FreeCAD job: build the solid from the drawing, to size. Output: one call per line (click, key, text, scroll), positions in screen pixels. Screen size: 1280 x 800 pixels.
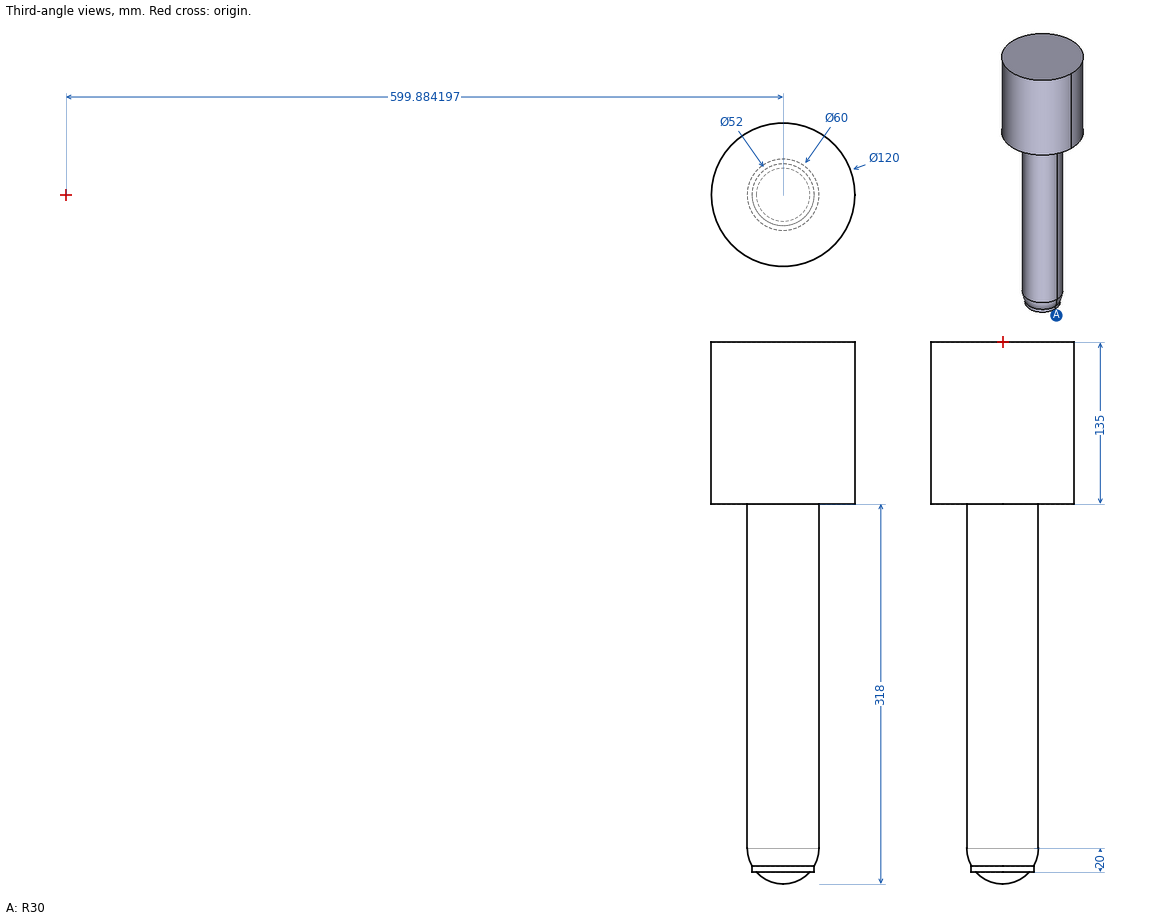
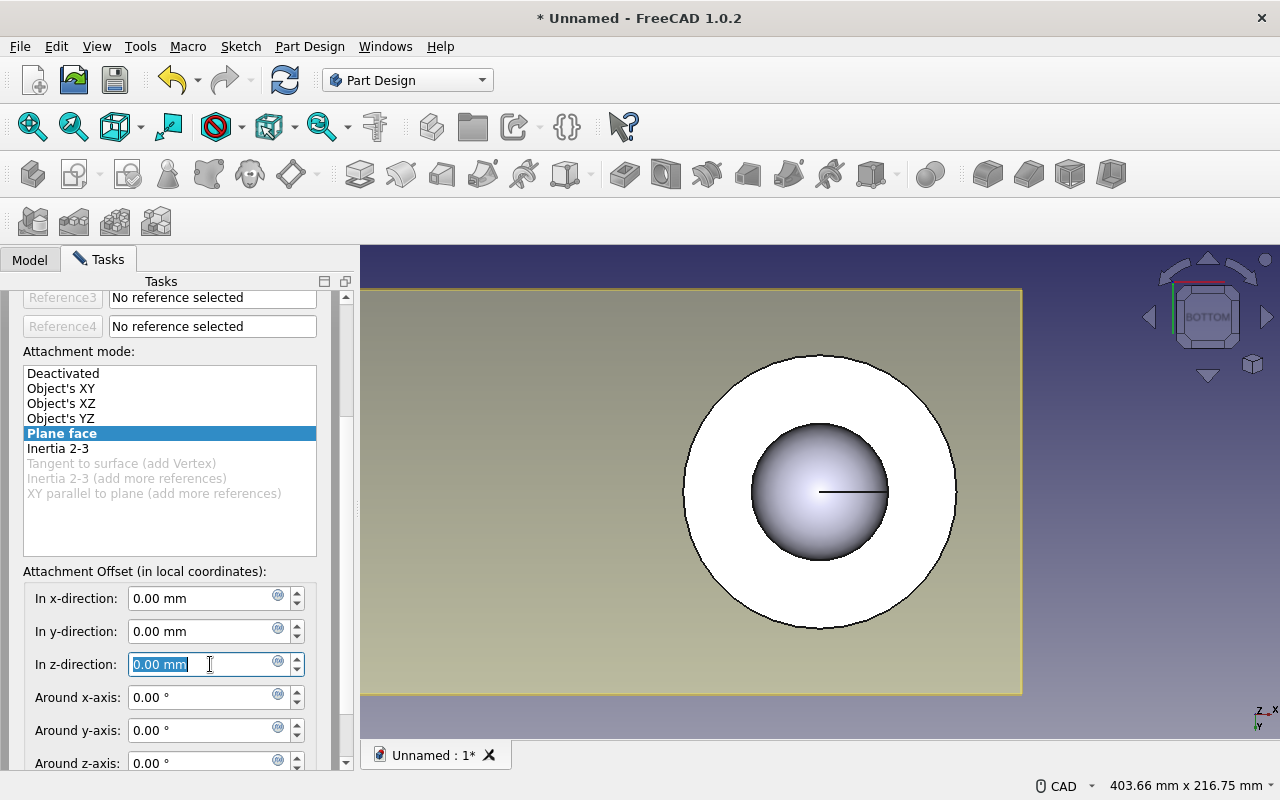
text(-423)
key(Tab)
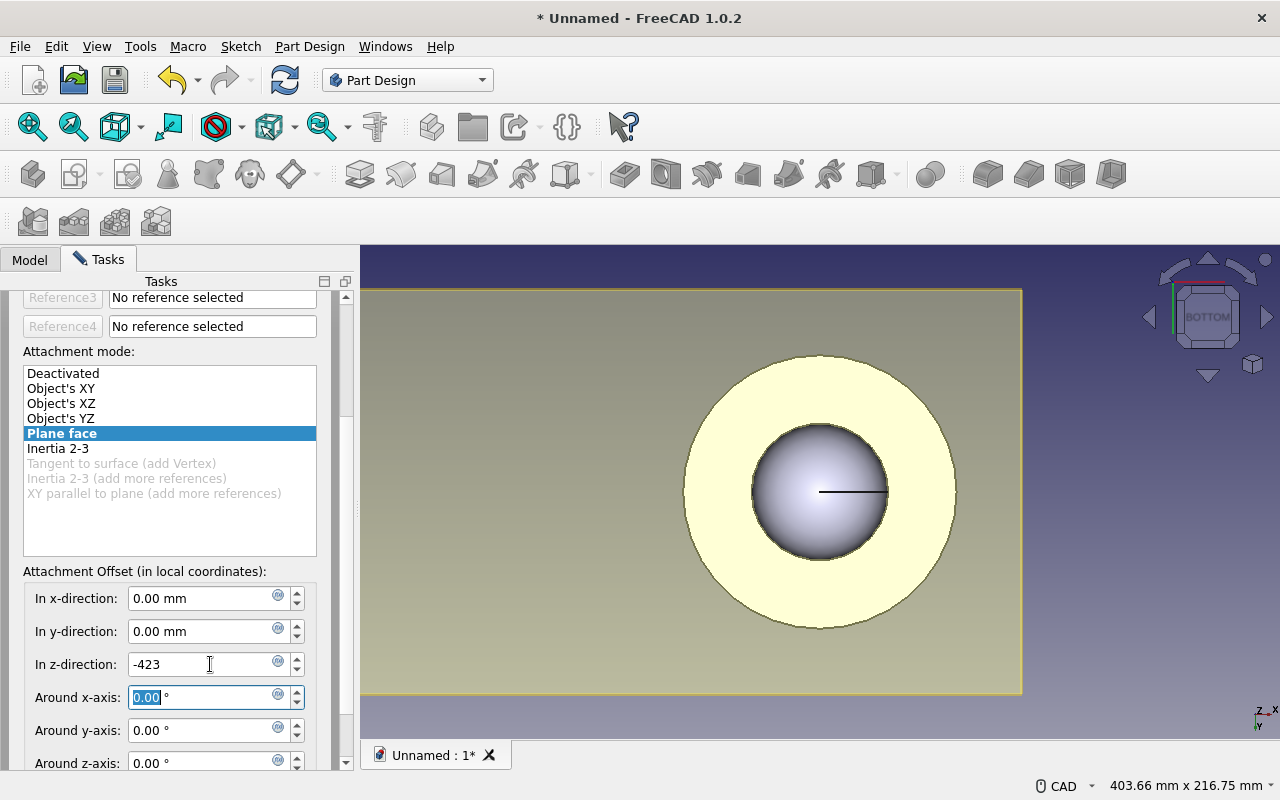
scroll(346, 530, up, 4)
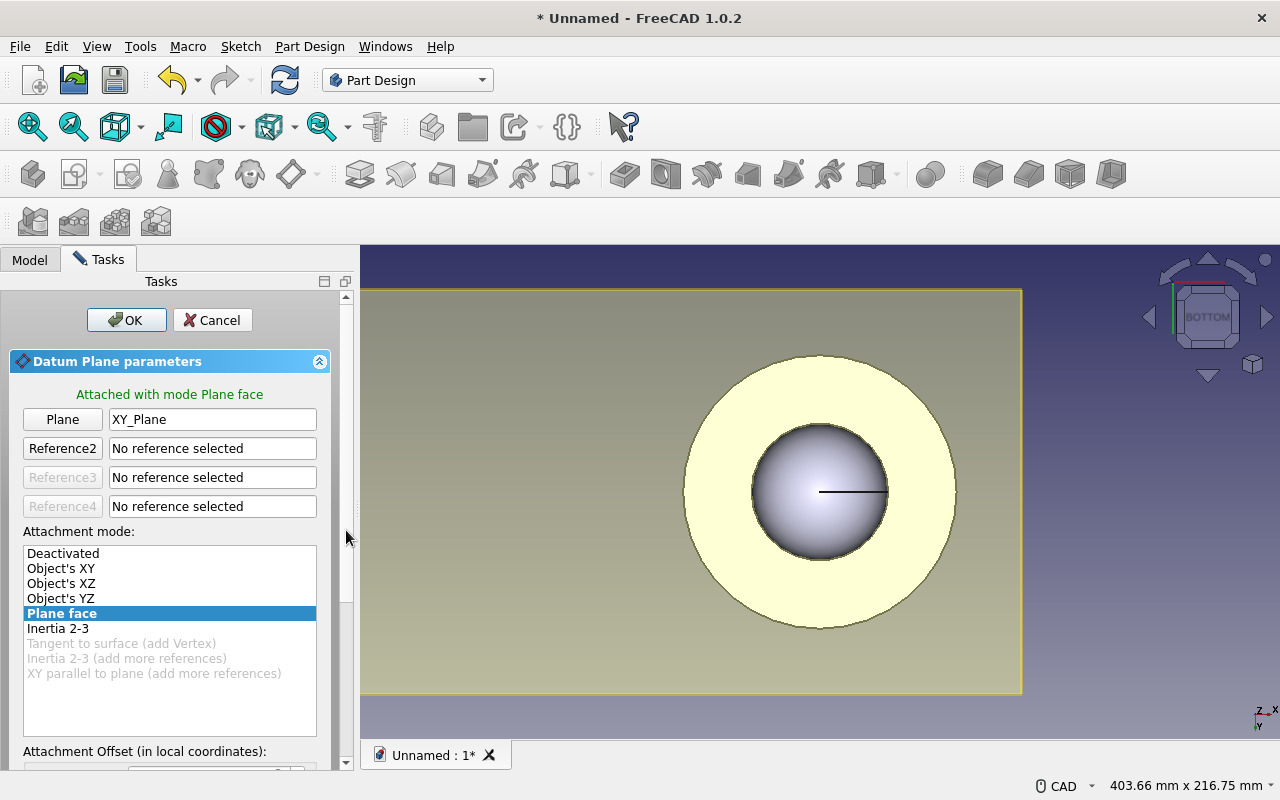
click(127, 320)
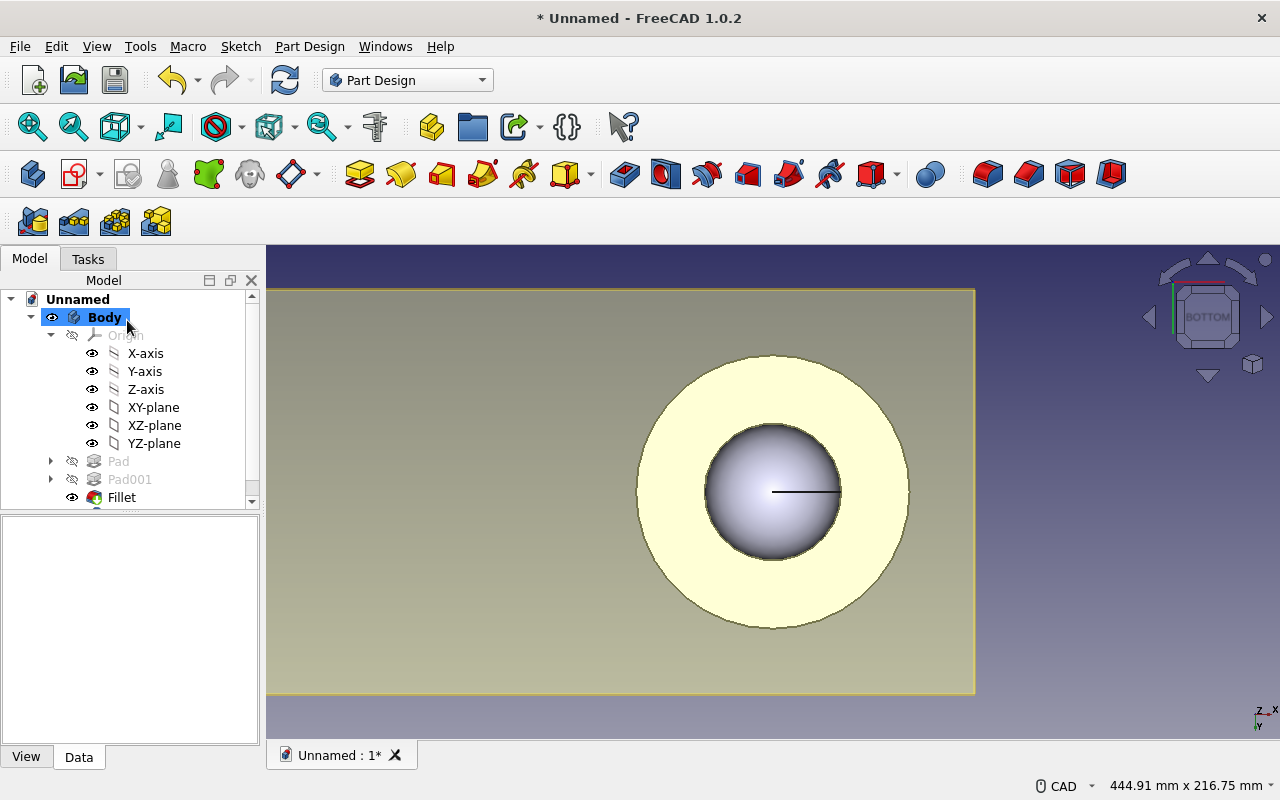
scroll(101, 403, down, 3)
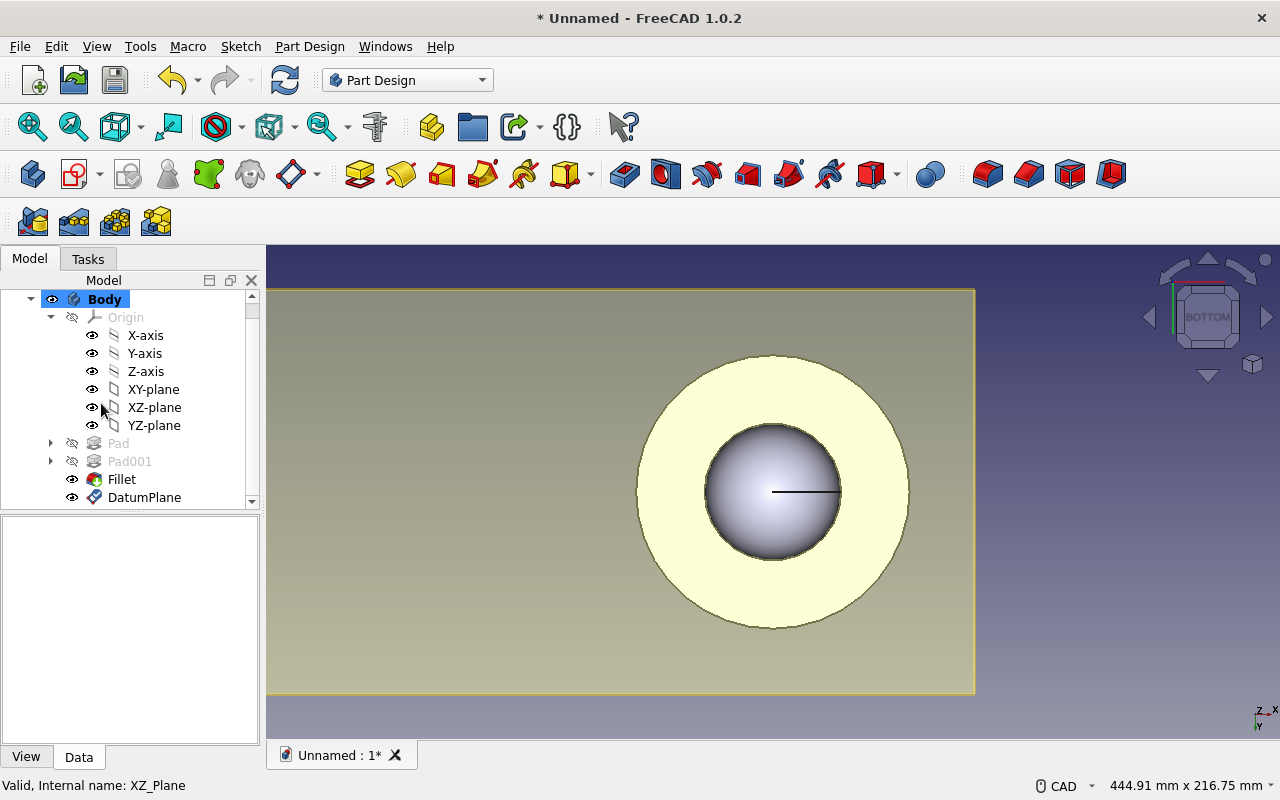
click(117, 497)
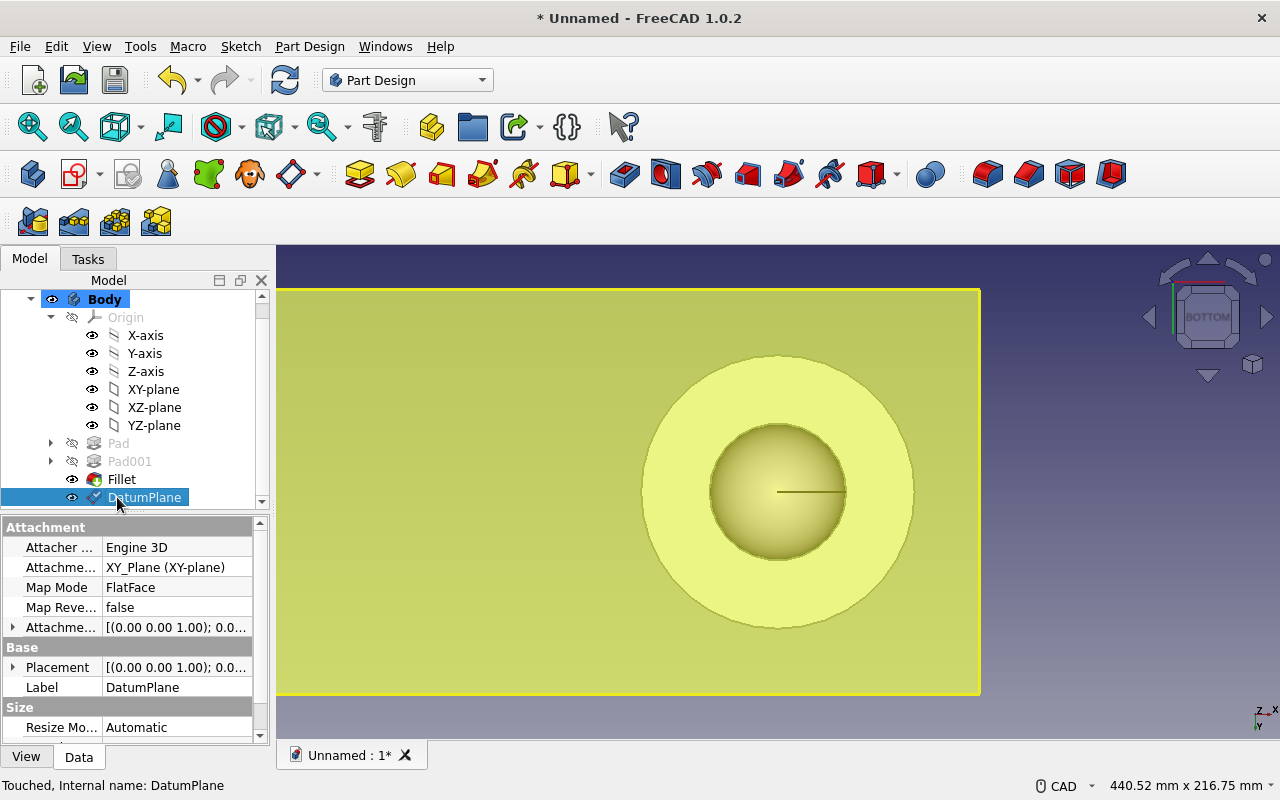
click(74, 174)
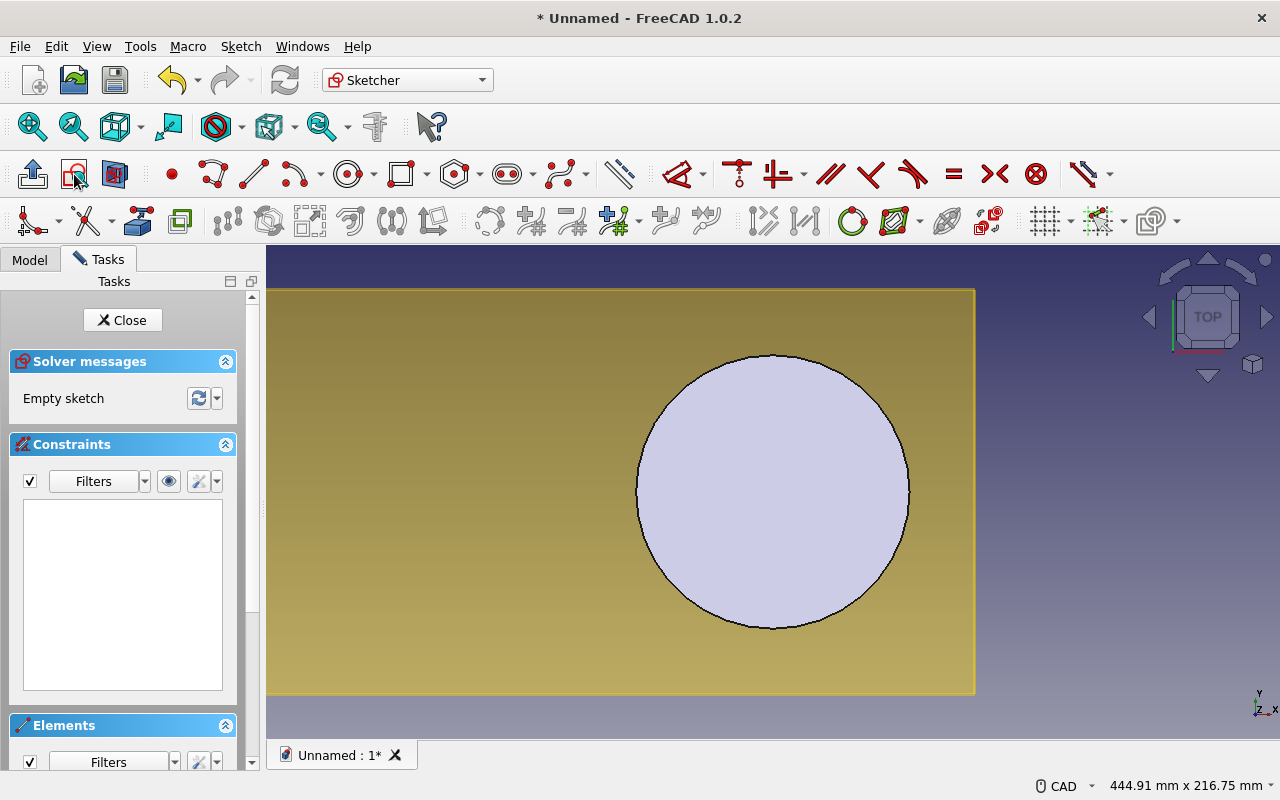
key(q)
key(s)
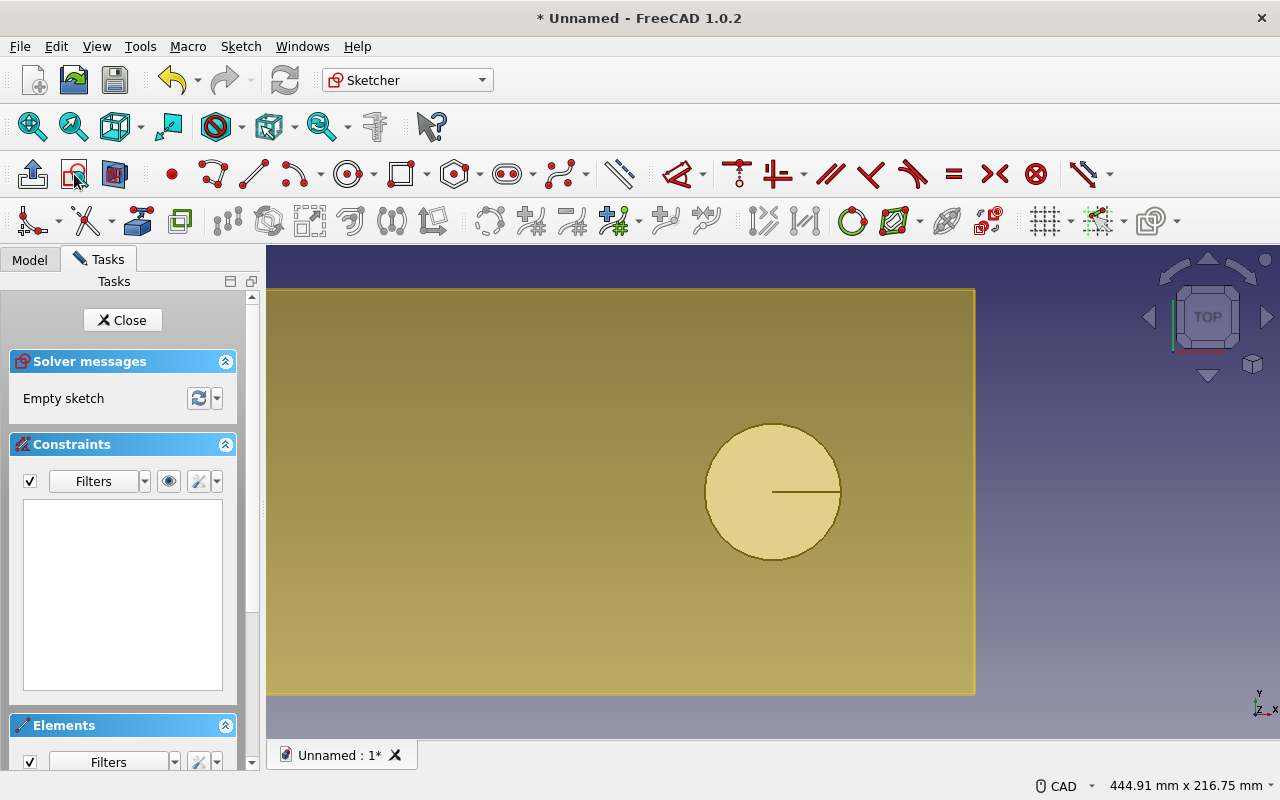
scroll(813, 492, up, 5)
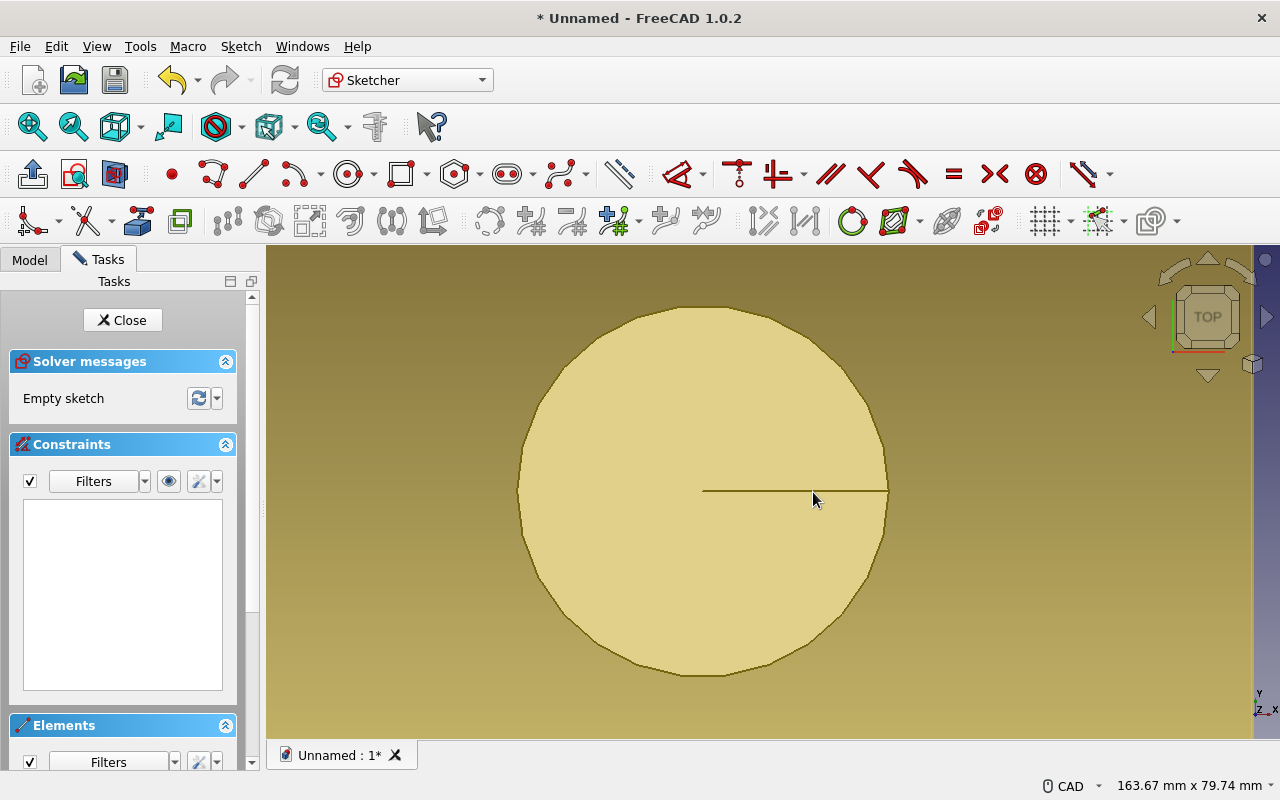
click(348, 174)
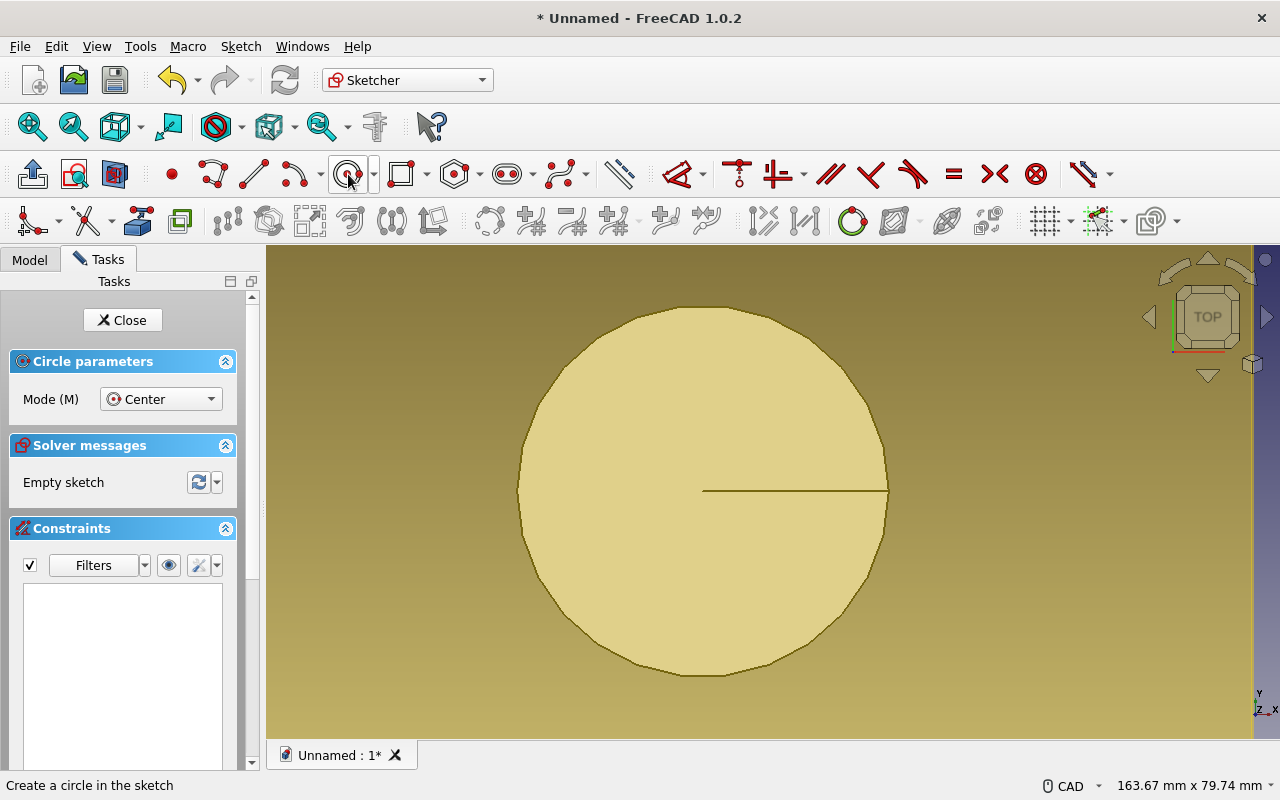
click(703, 491)
move(817, 377)